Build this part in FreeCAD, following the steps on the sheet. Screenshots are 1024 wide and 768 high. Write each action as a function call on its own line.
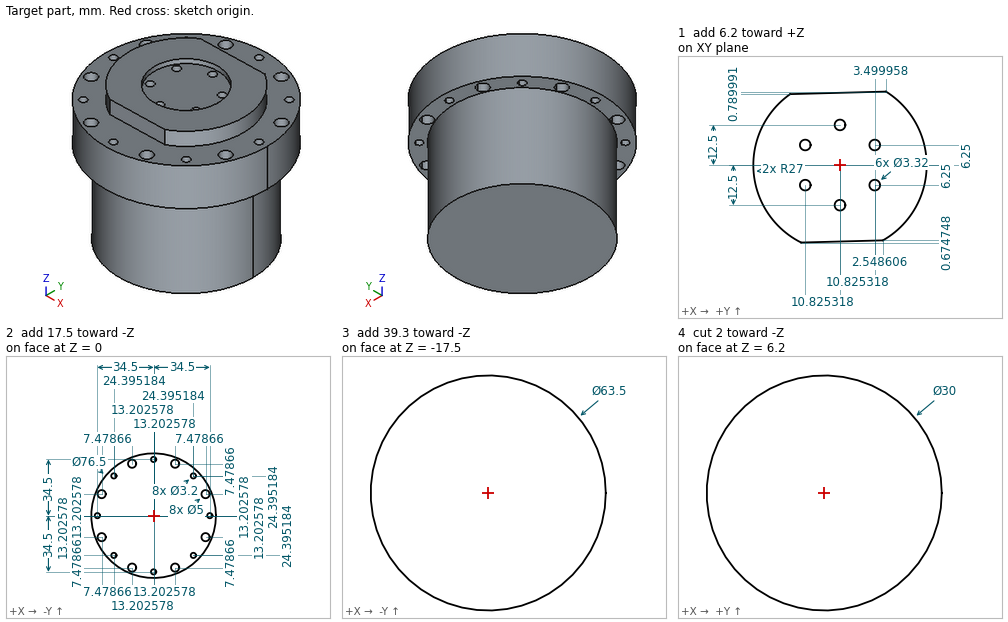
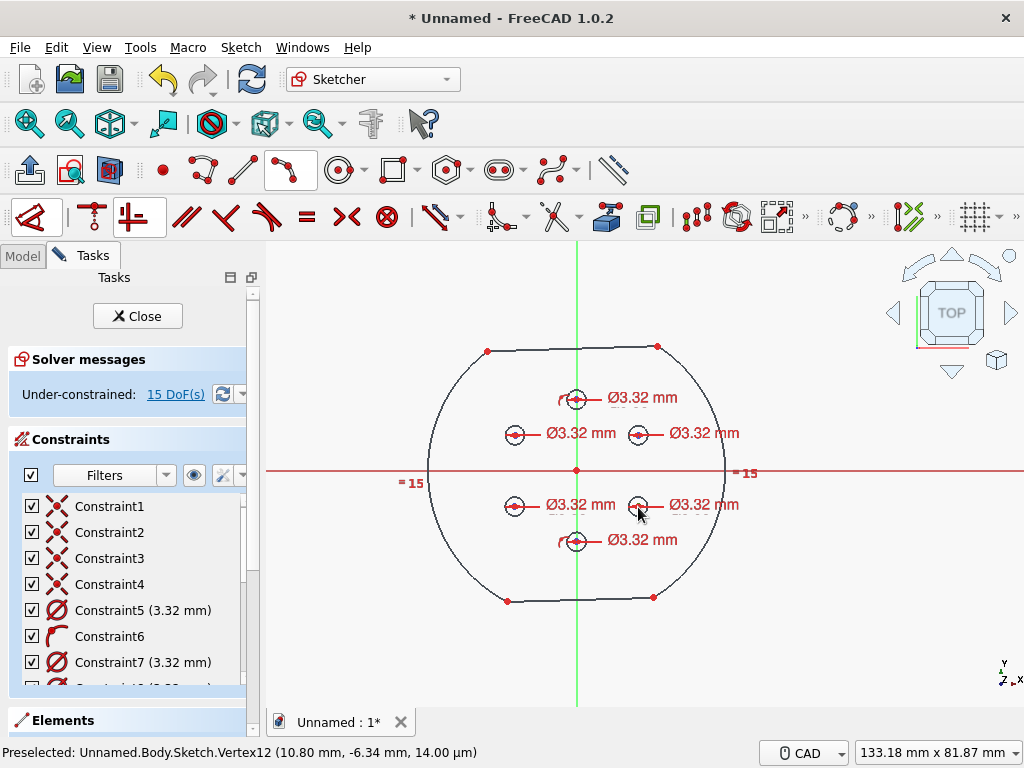
click(515, 507)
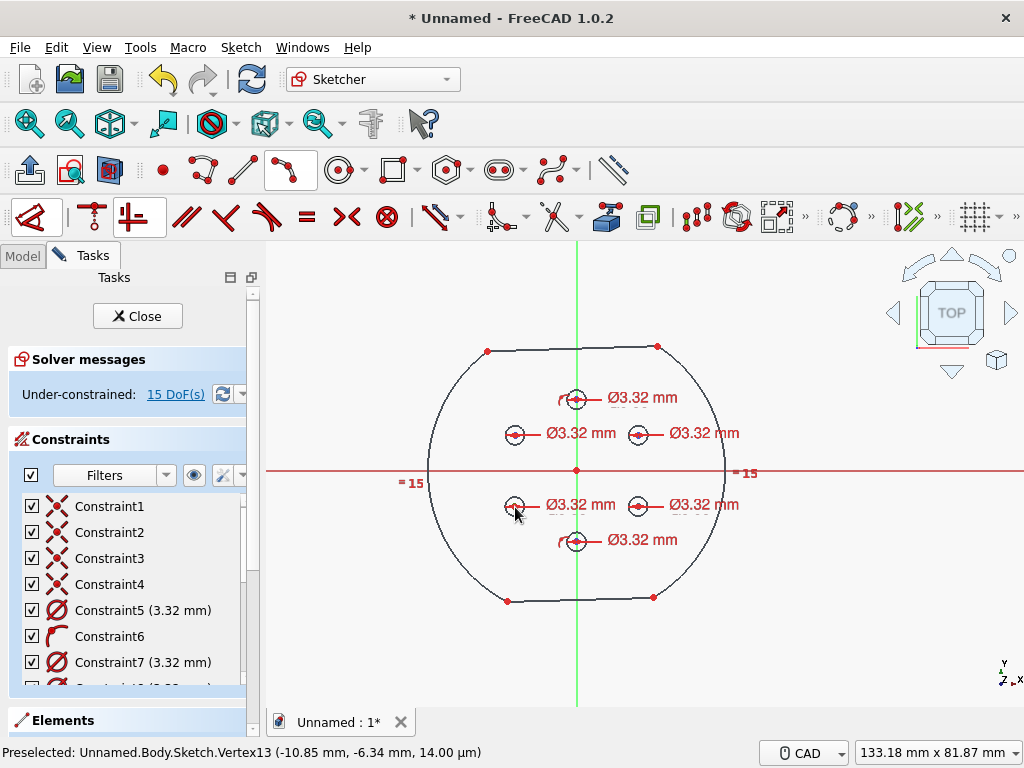
click(160, 218)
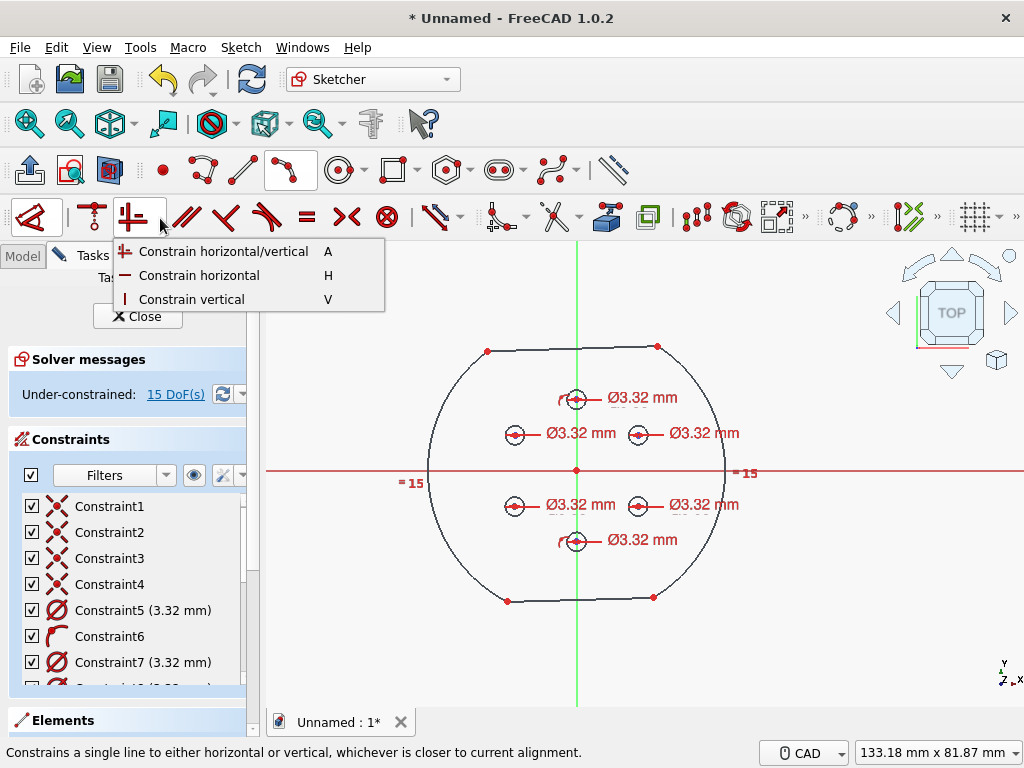
click(249, 275)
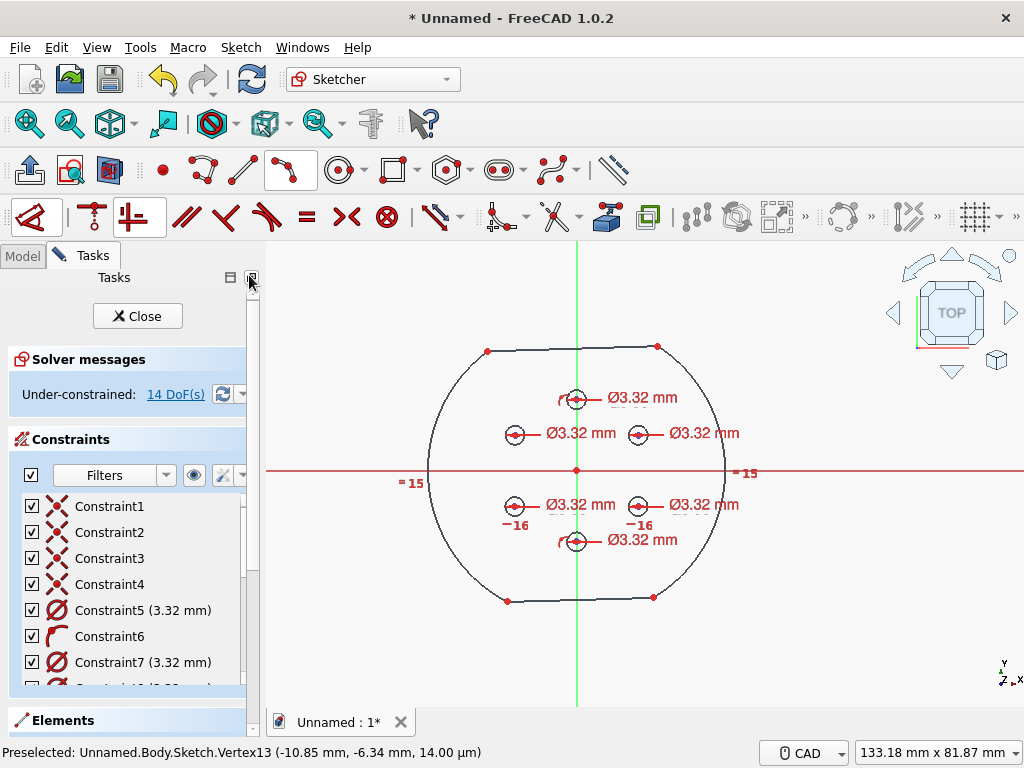
click(638, 507)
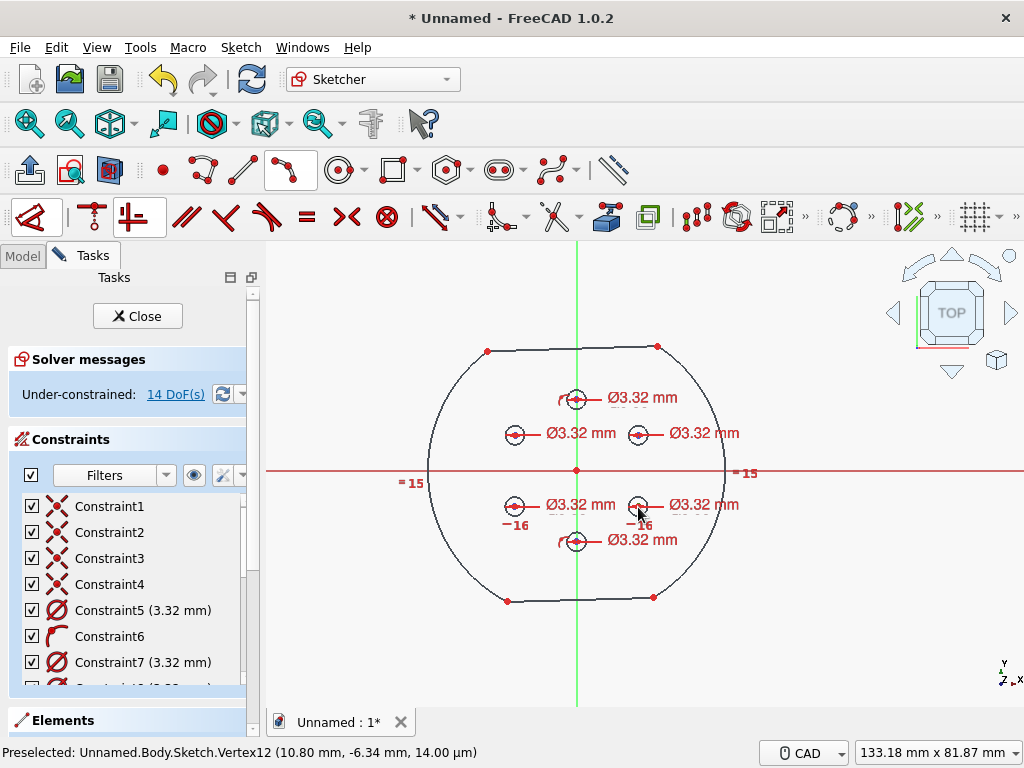
click(638, 435)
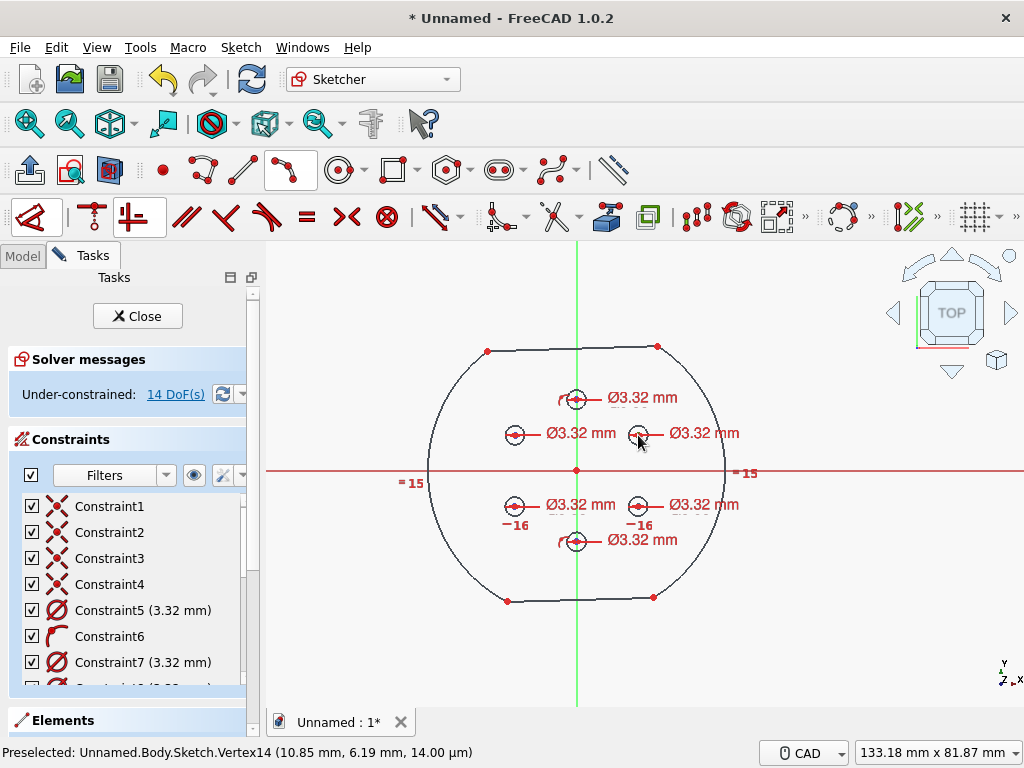
key(v)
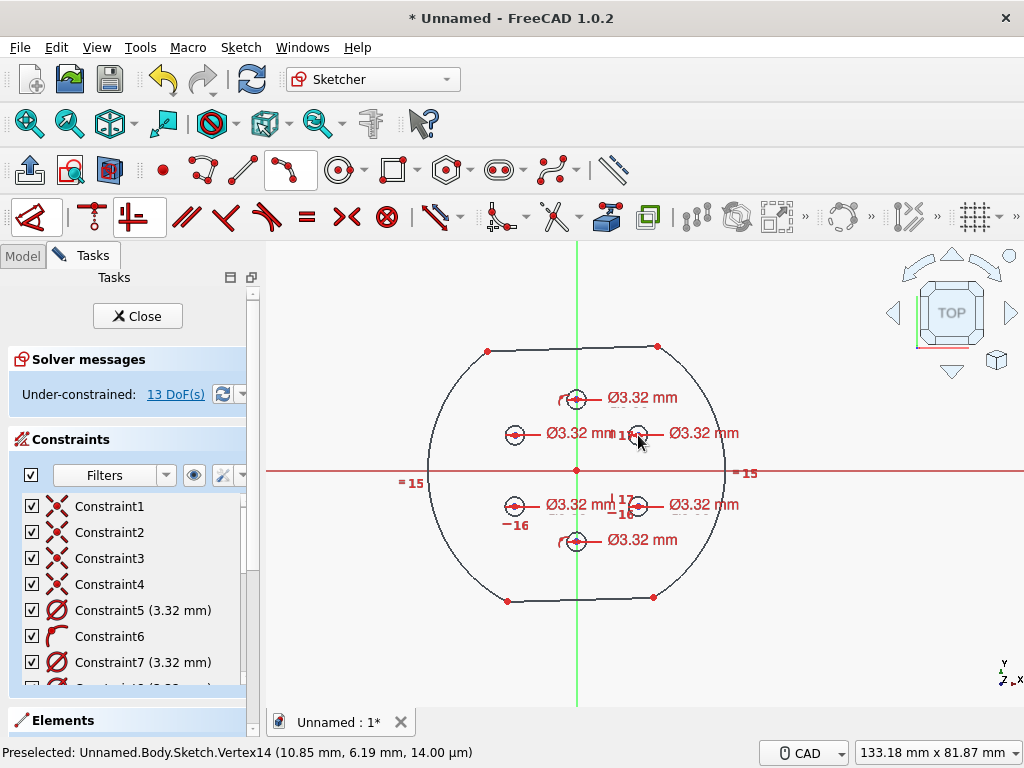
click(515, 507)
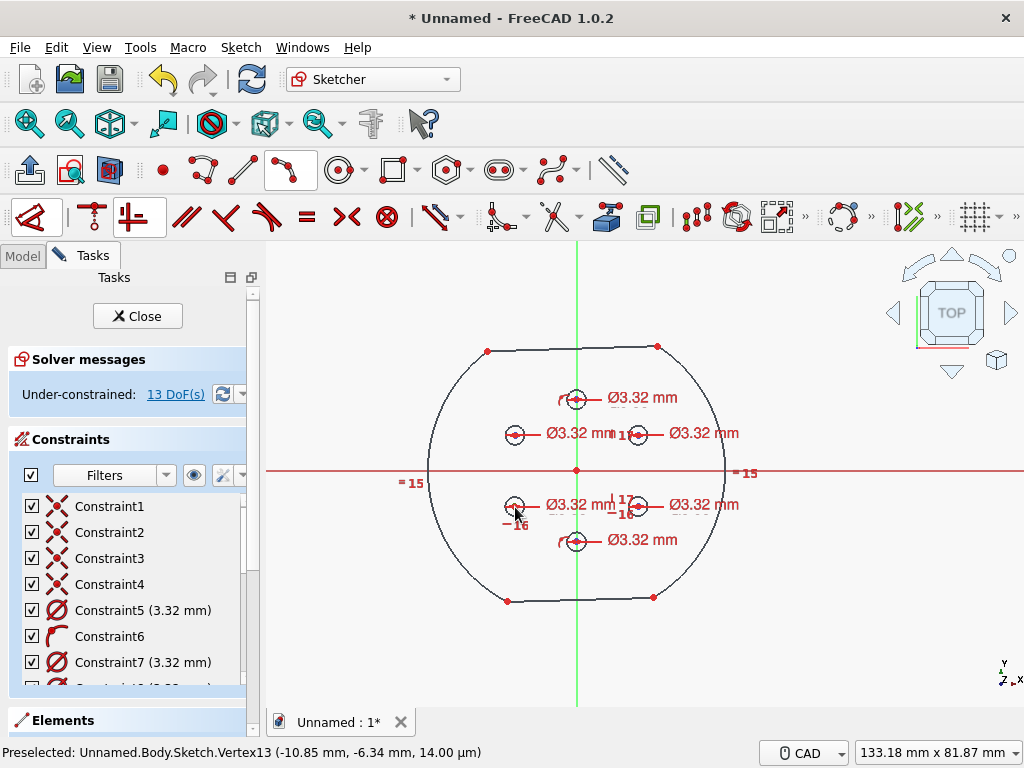
click(515, 435)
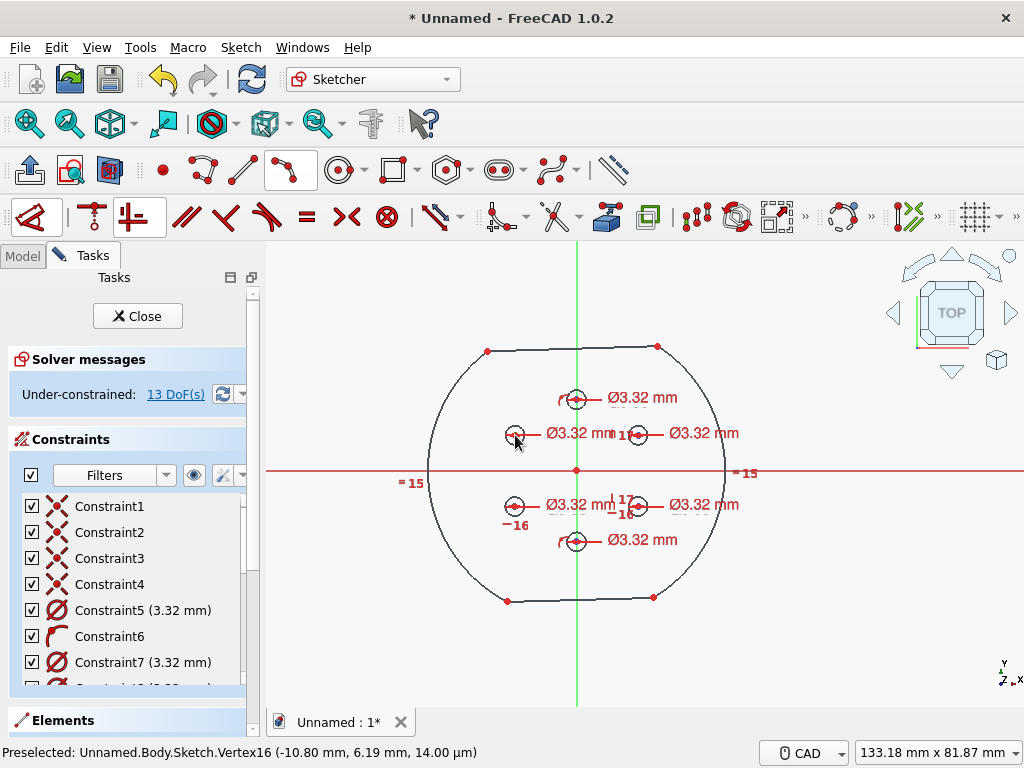
click(160, 218)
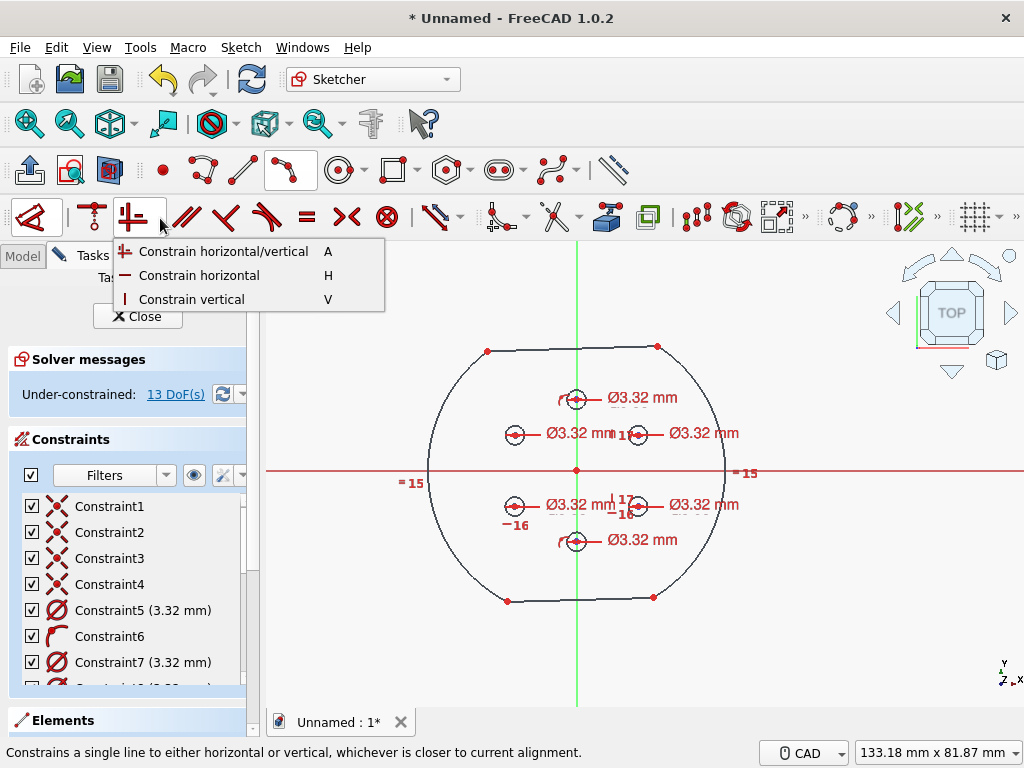
click(249, 299)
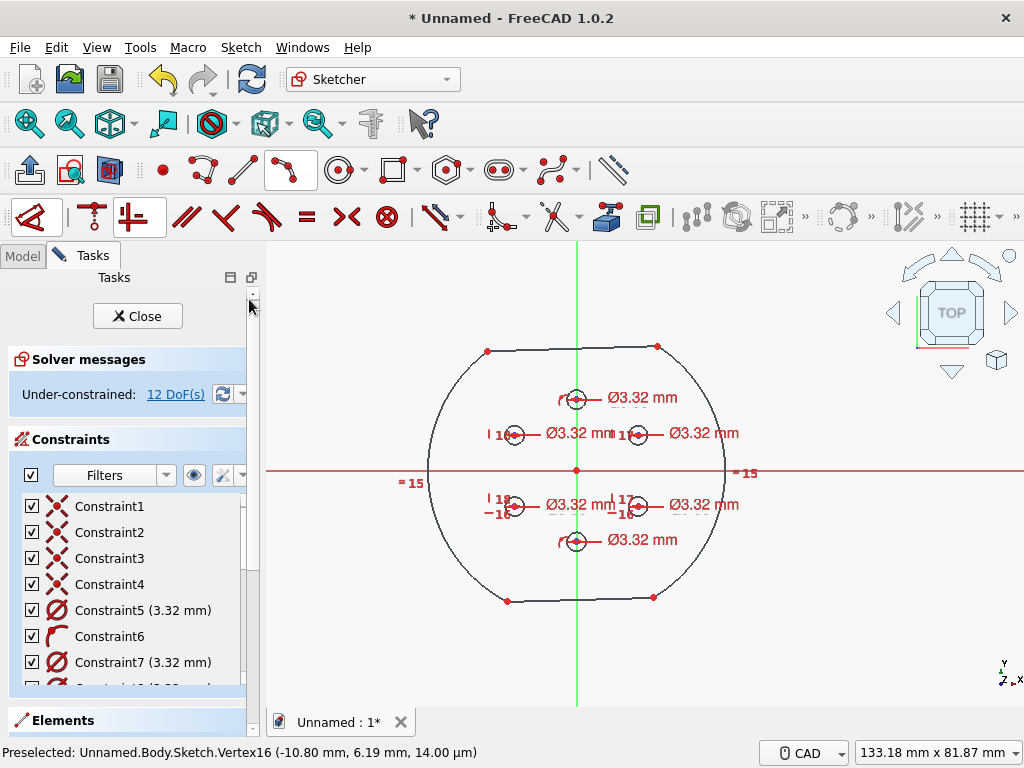
click(638, 435)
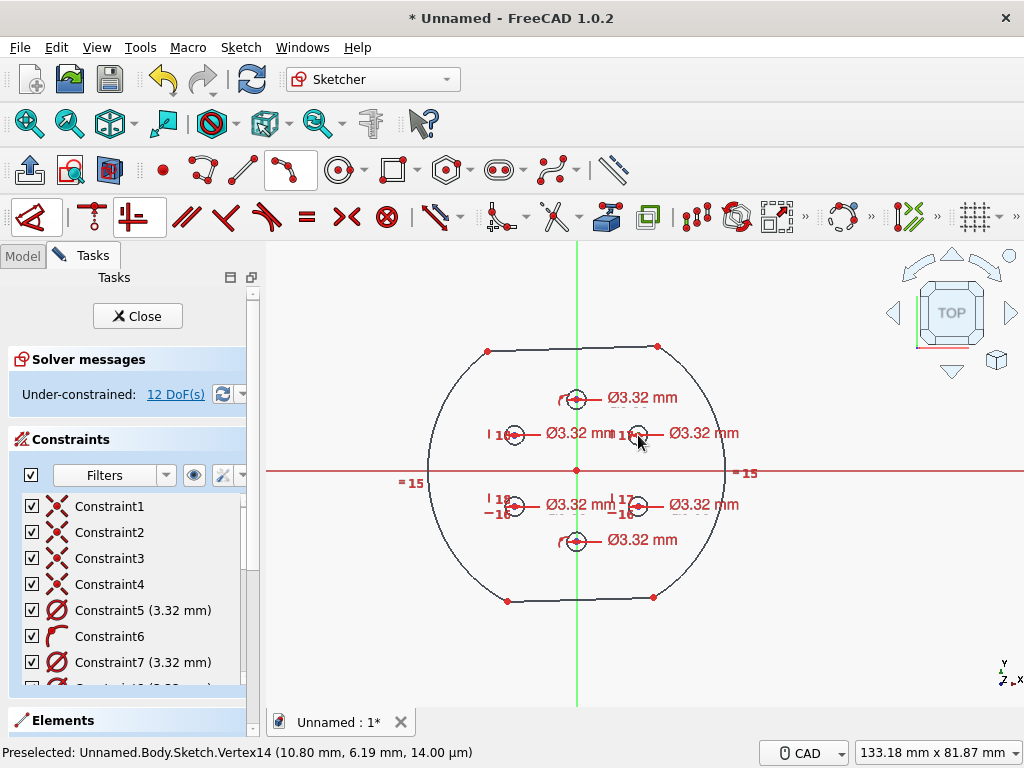
click(515, 435)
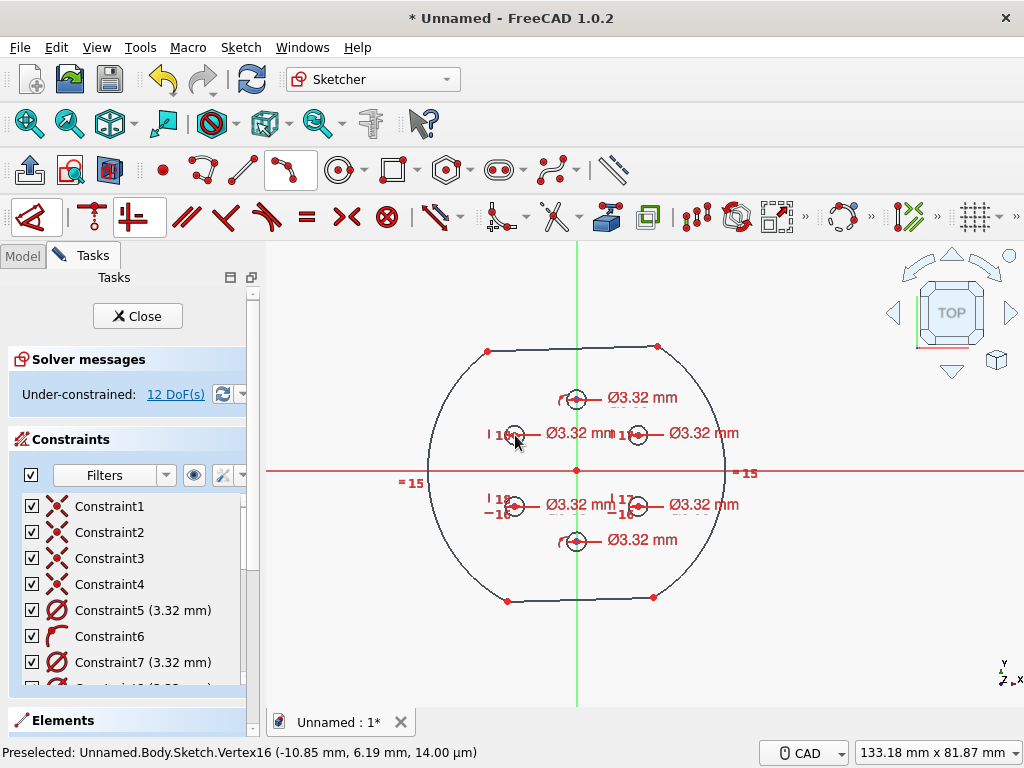
key(h)